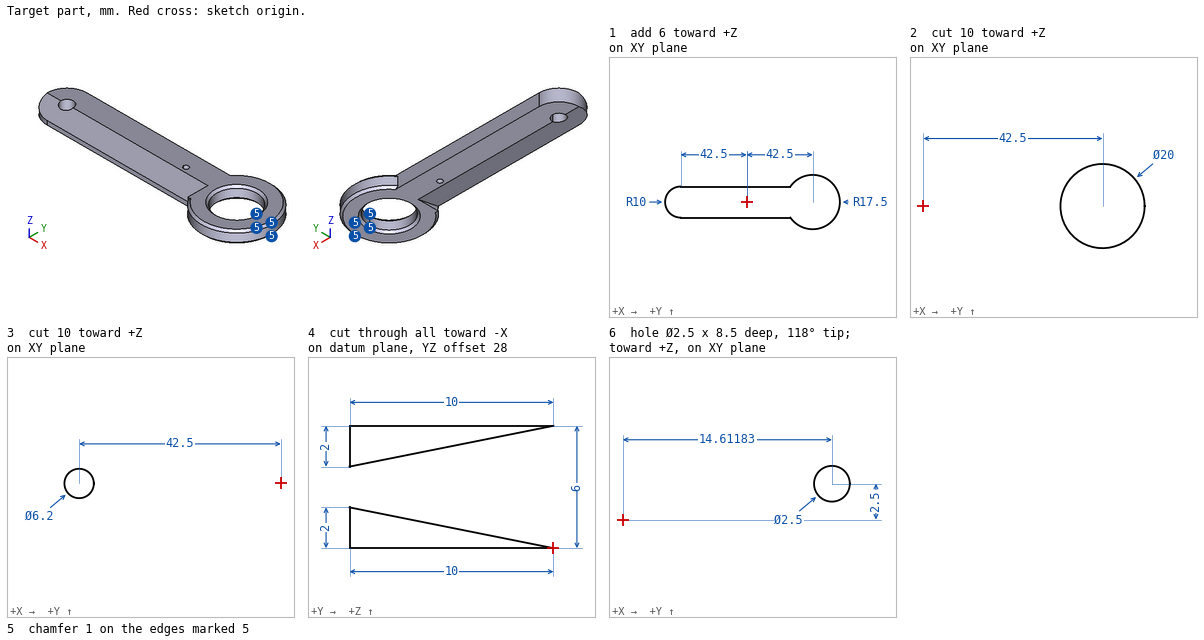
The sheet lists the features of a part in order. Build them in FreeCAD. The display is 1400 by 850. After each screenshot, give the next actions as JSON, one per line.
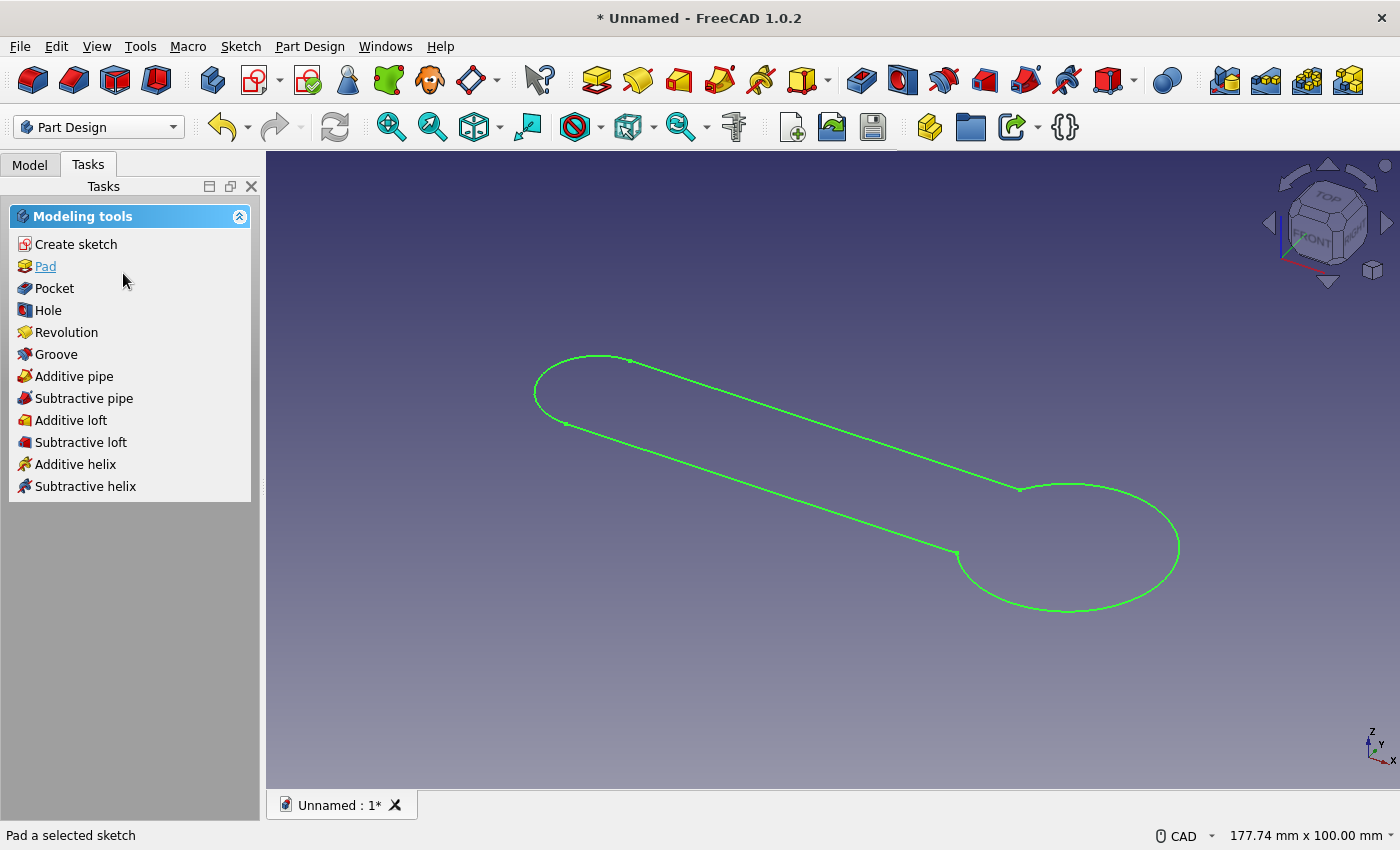
{"action": "left_click", "coordinate": [597, 80]}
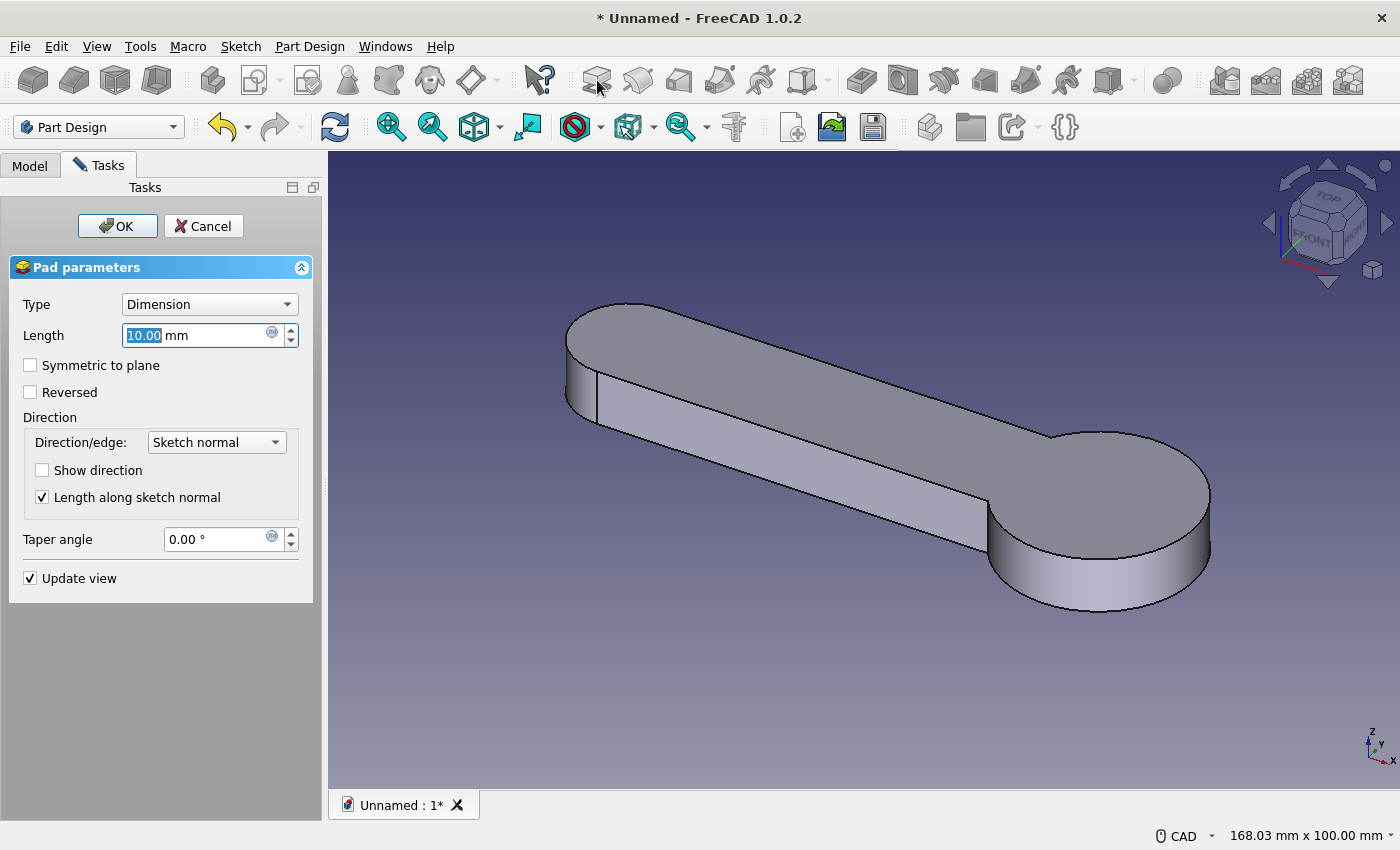
{"action": "type", "text": "6"}
{"action": "key", "text": "Tab"}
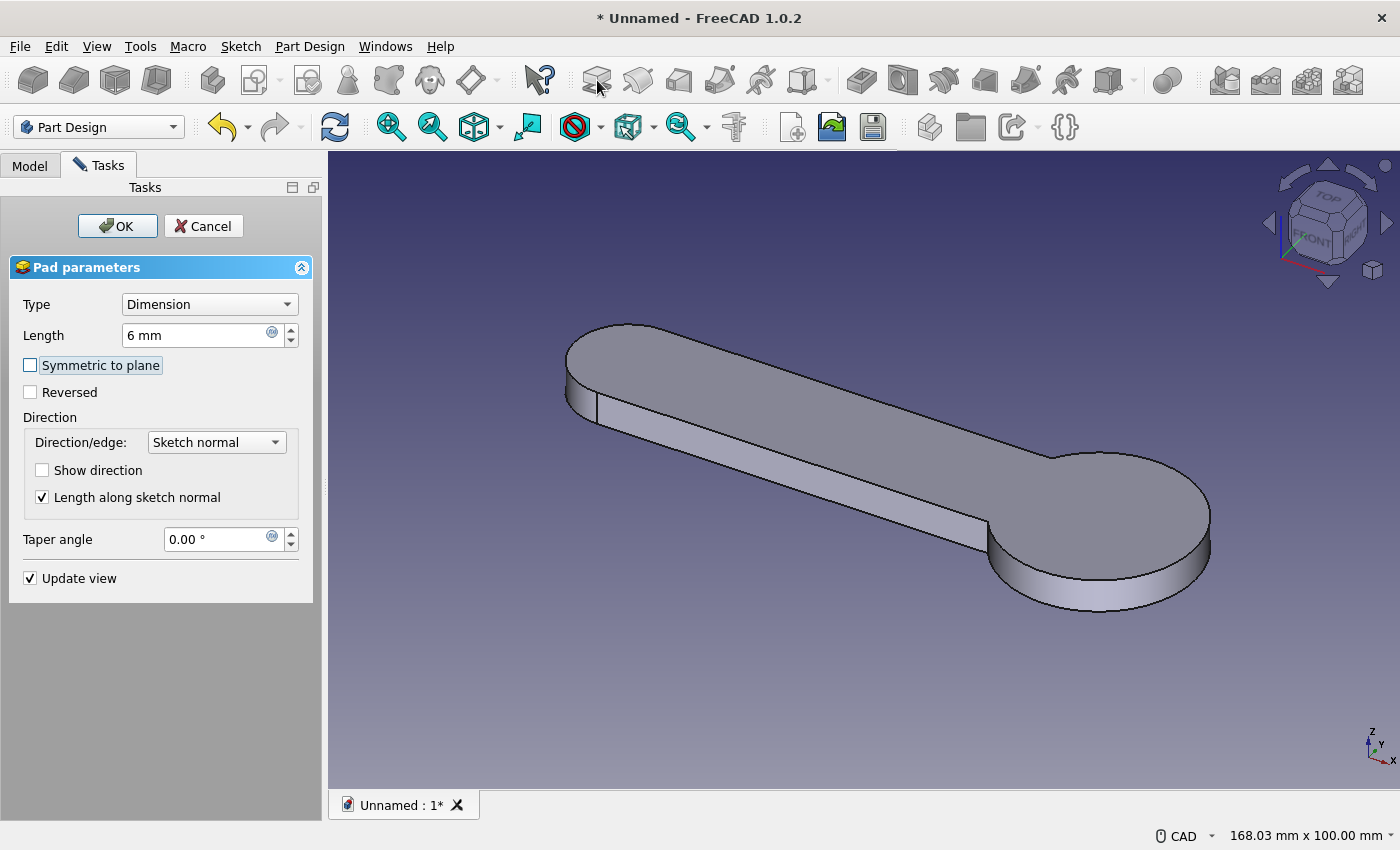
{"action": "left_click", "coordinate": [118, 226]}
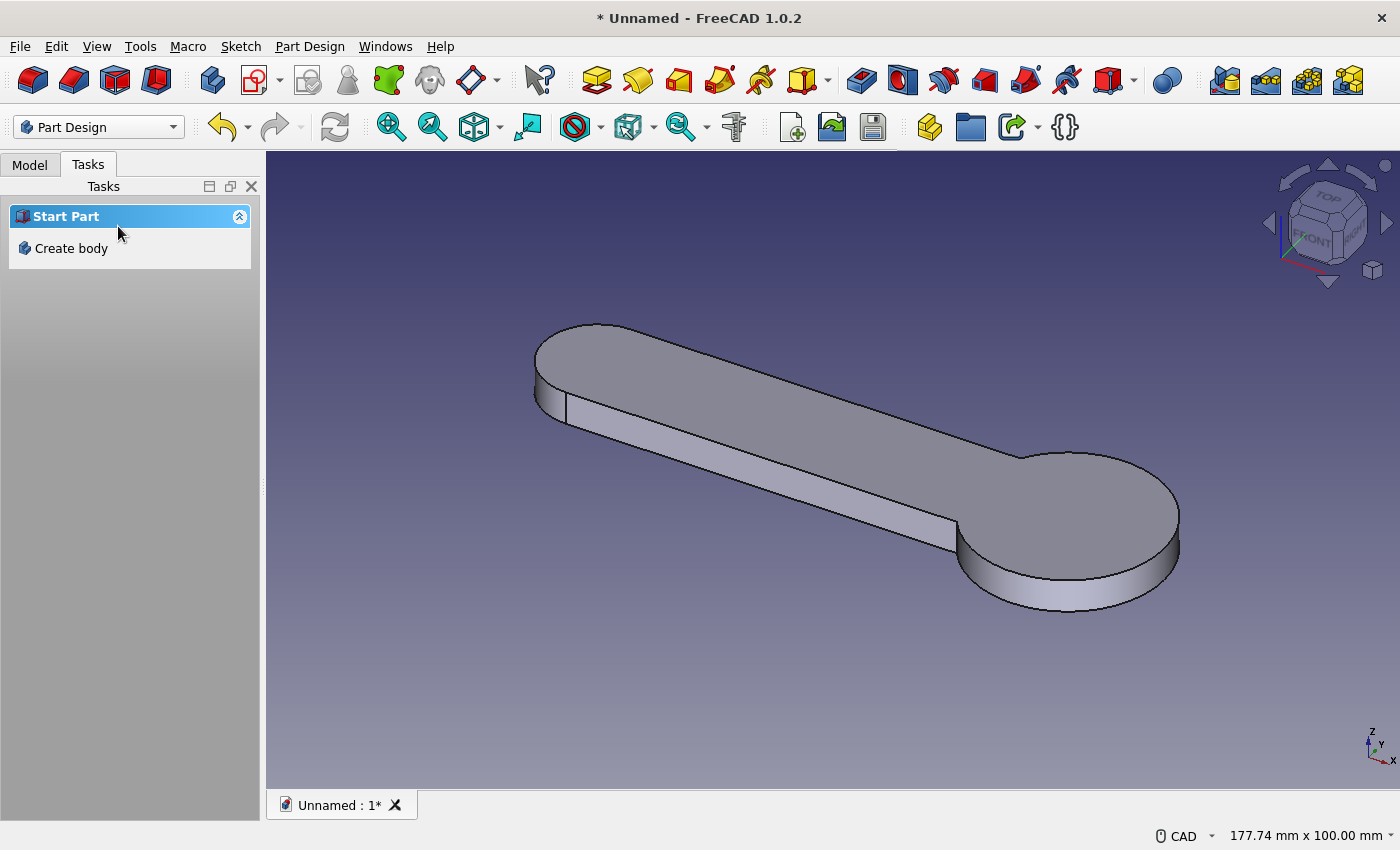
{"action": "left_click", "coordinate": [254, 80]}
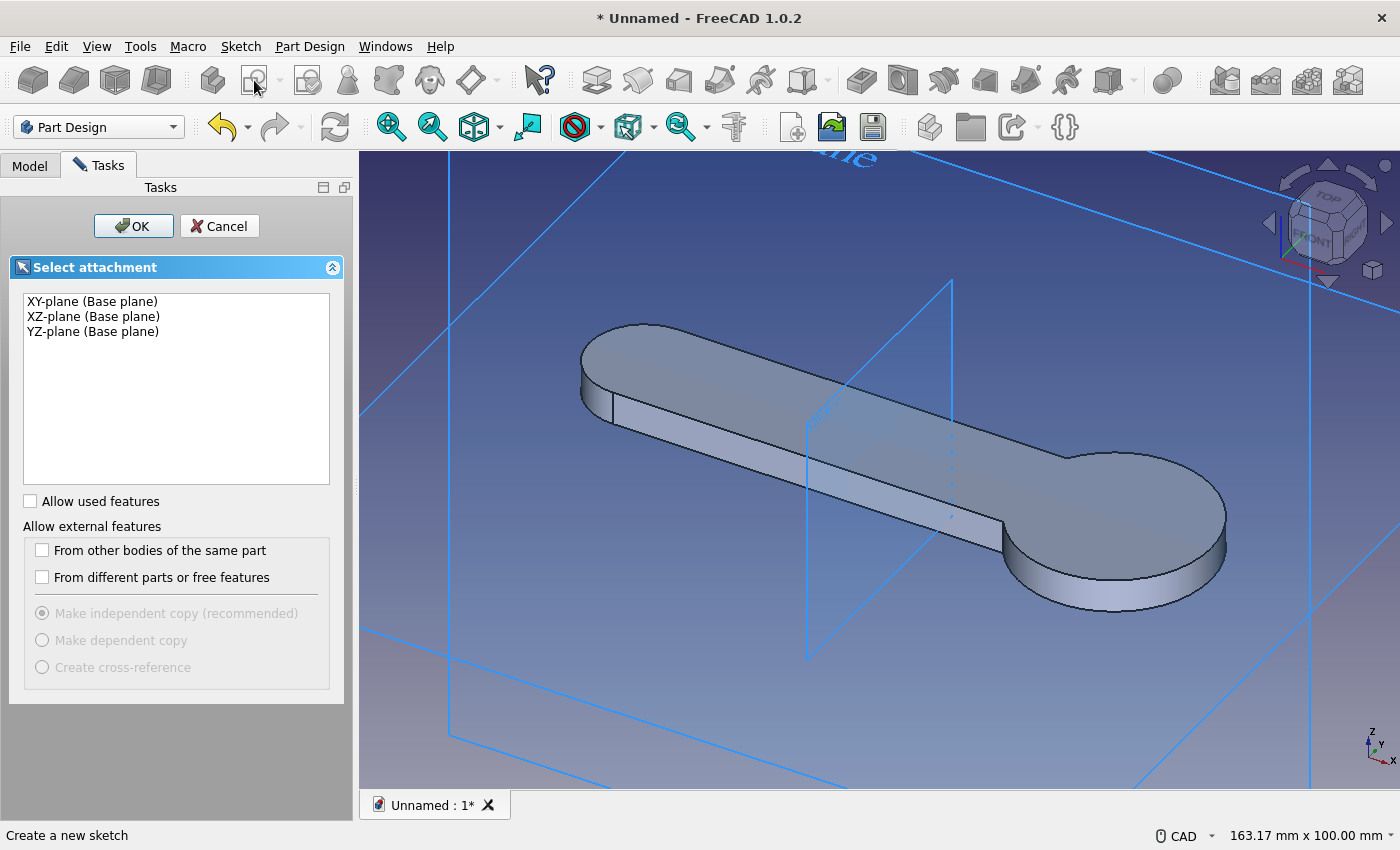
{"action": "left_click", "coordinate": [84, 302]}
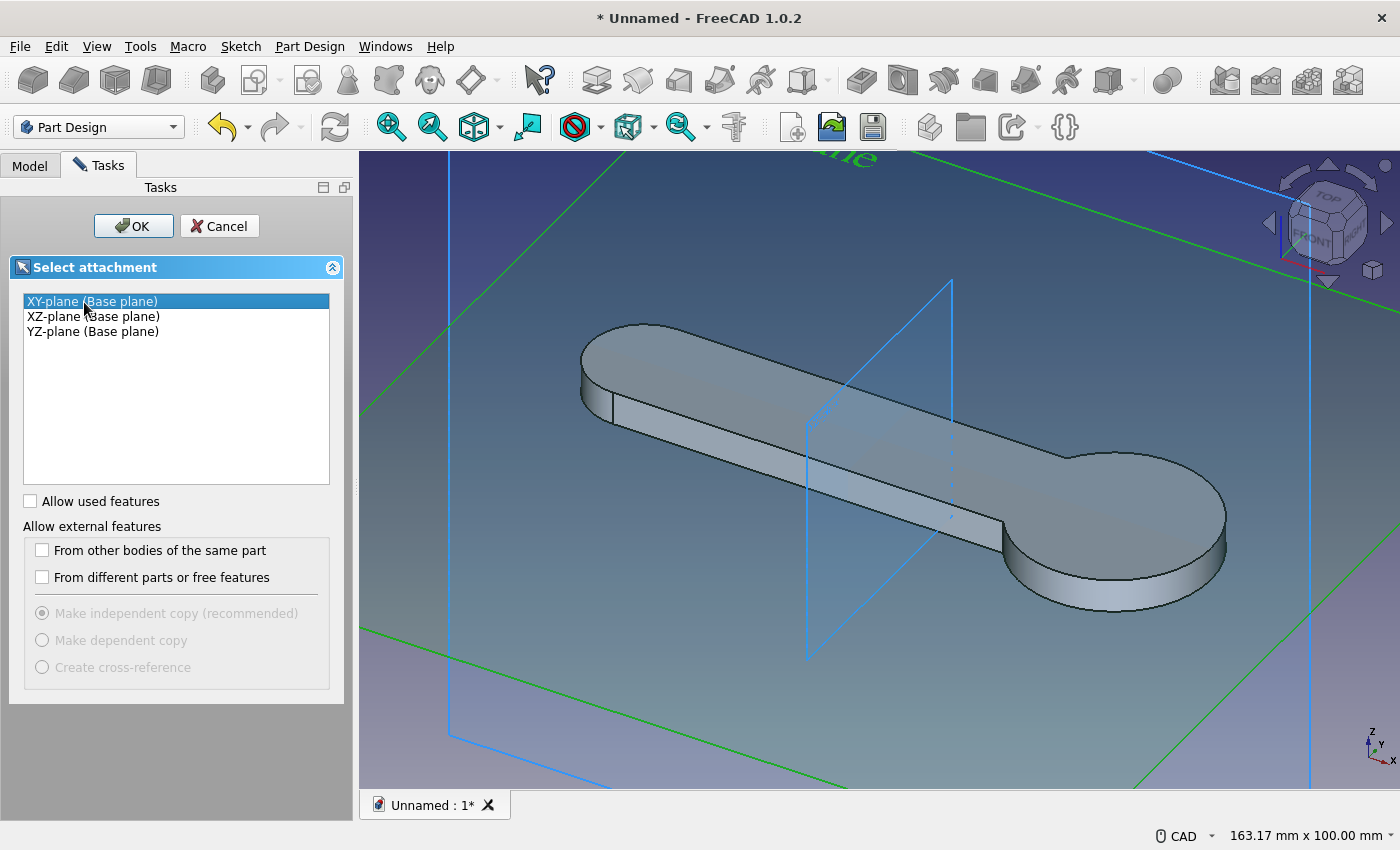
{"action": "left_click", "coordinate": [134, 226]}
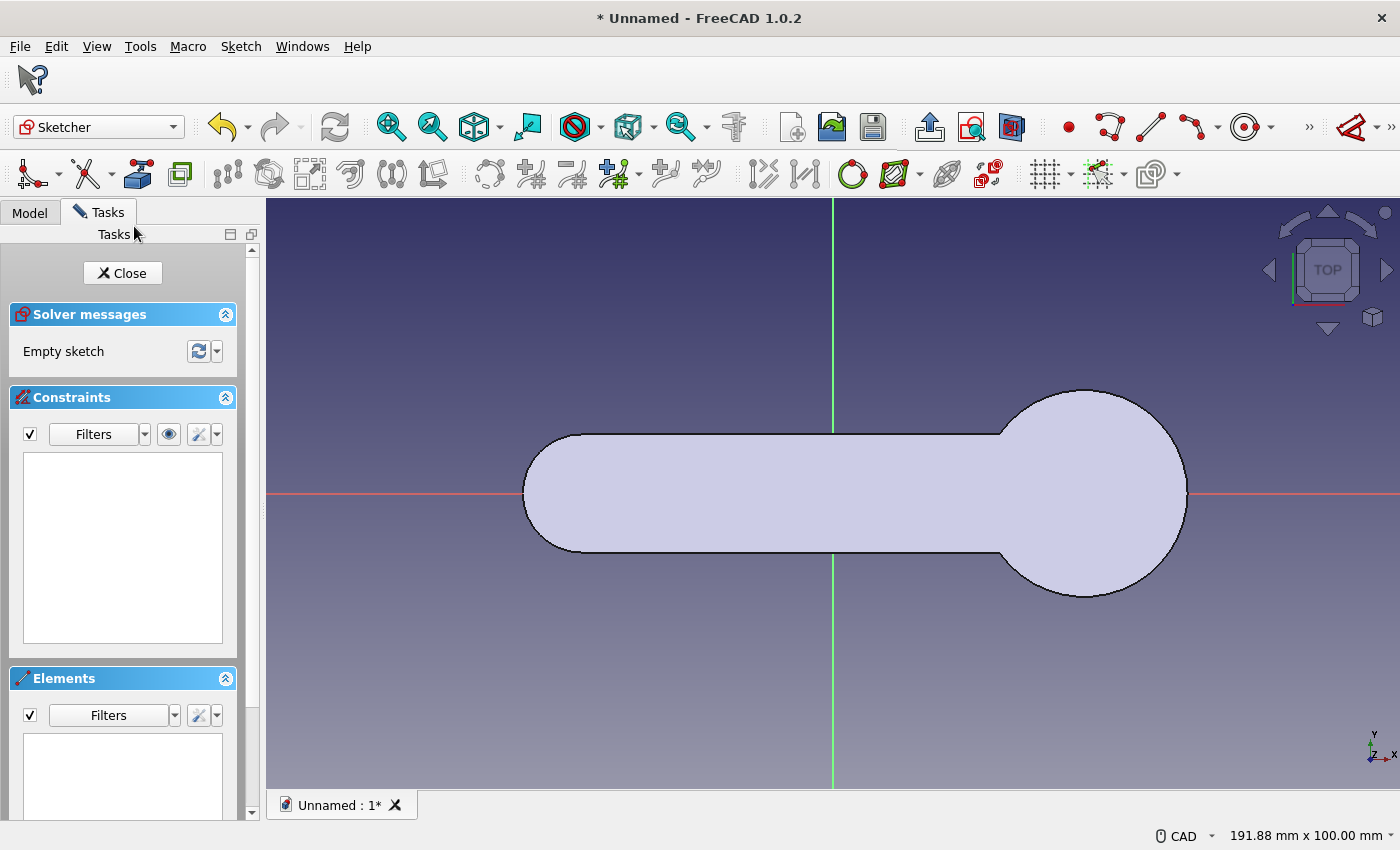
{"action": "left_click", "coordinate": [1012, 128]}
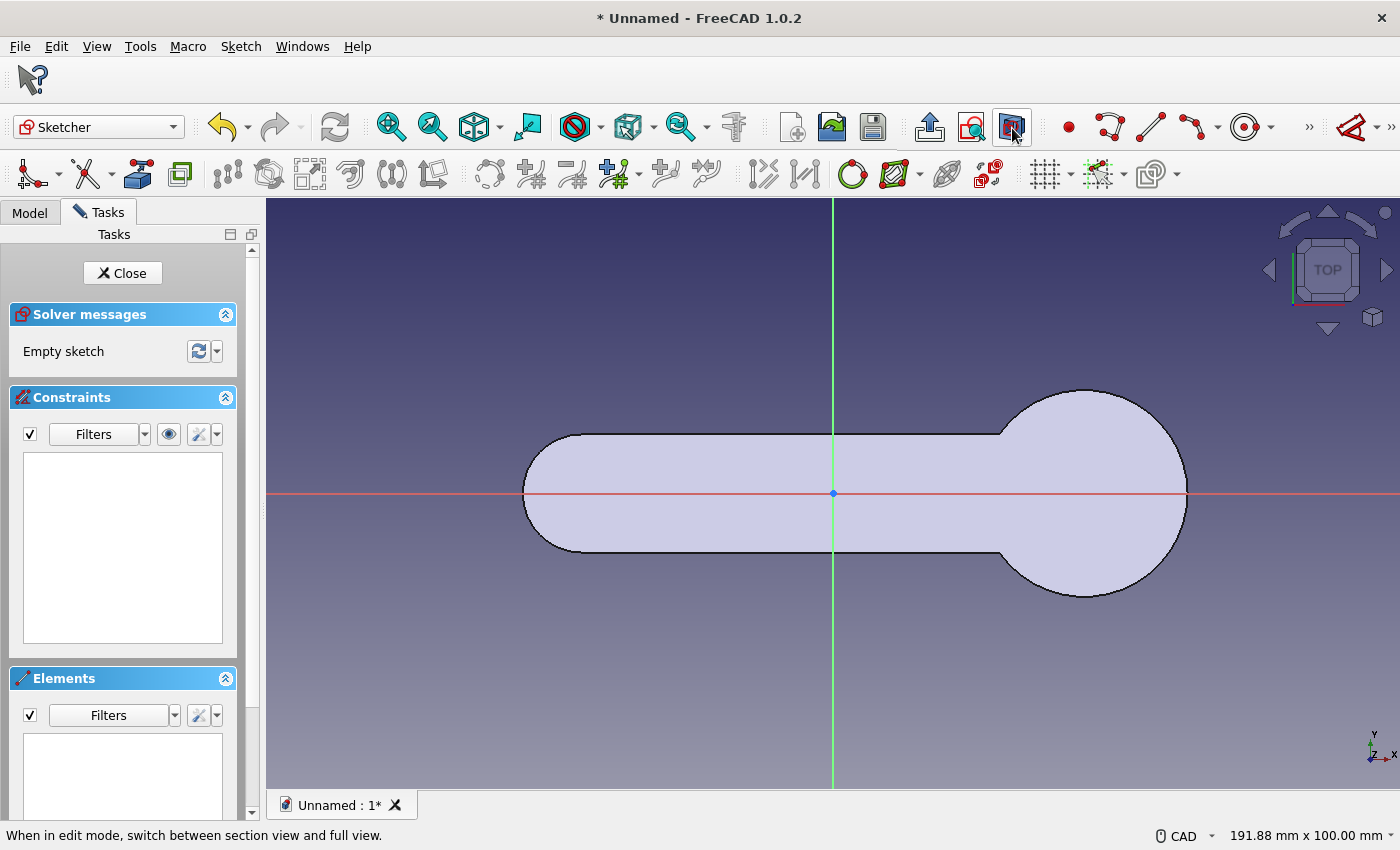
{"action": "scroll", "coordinate": [1222, 494], "scroll_direction": "up", "scroll_amount": 6}